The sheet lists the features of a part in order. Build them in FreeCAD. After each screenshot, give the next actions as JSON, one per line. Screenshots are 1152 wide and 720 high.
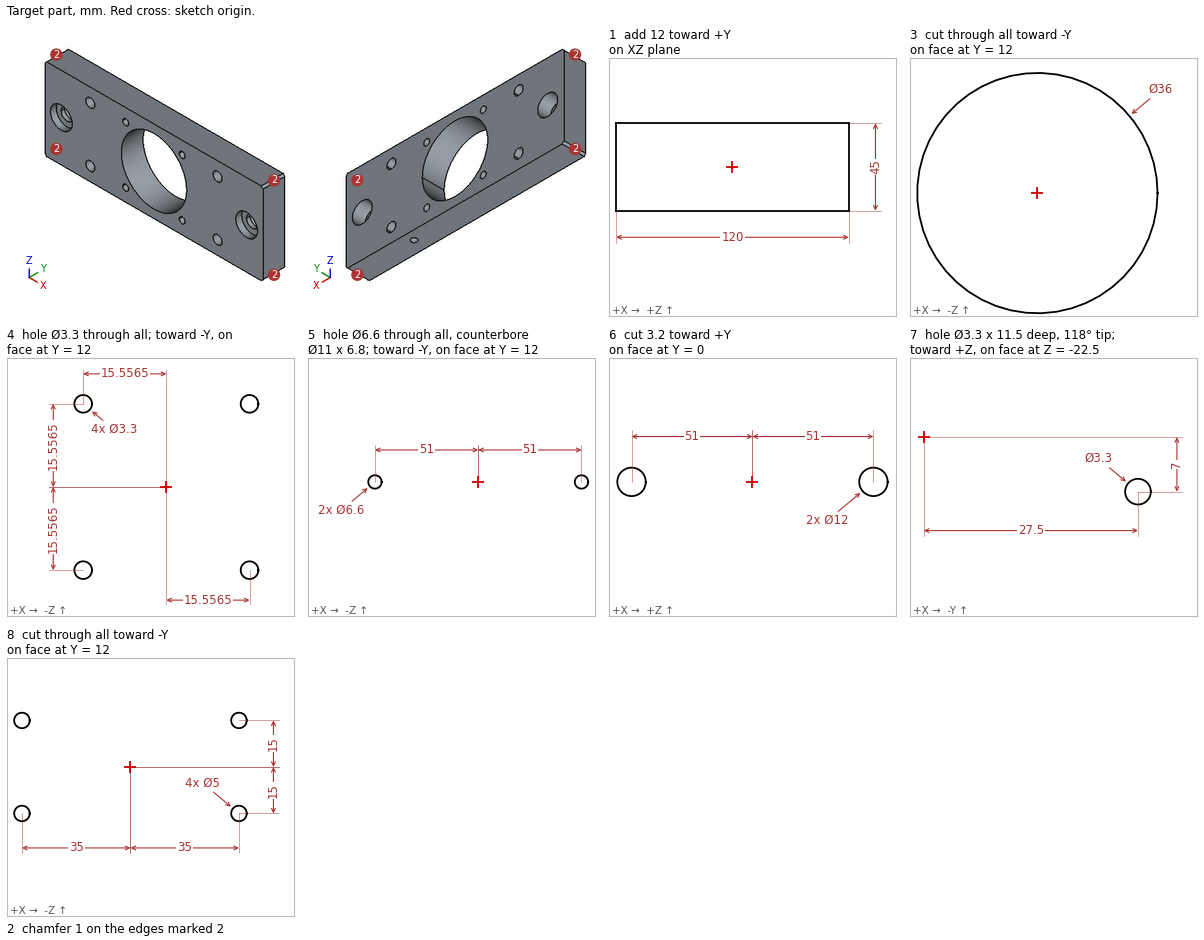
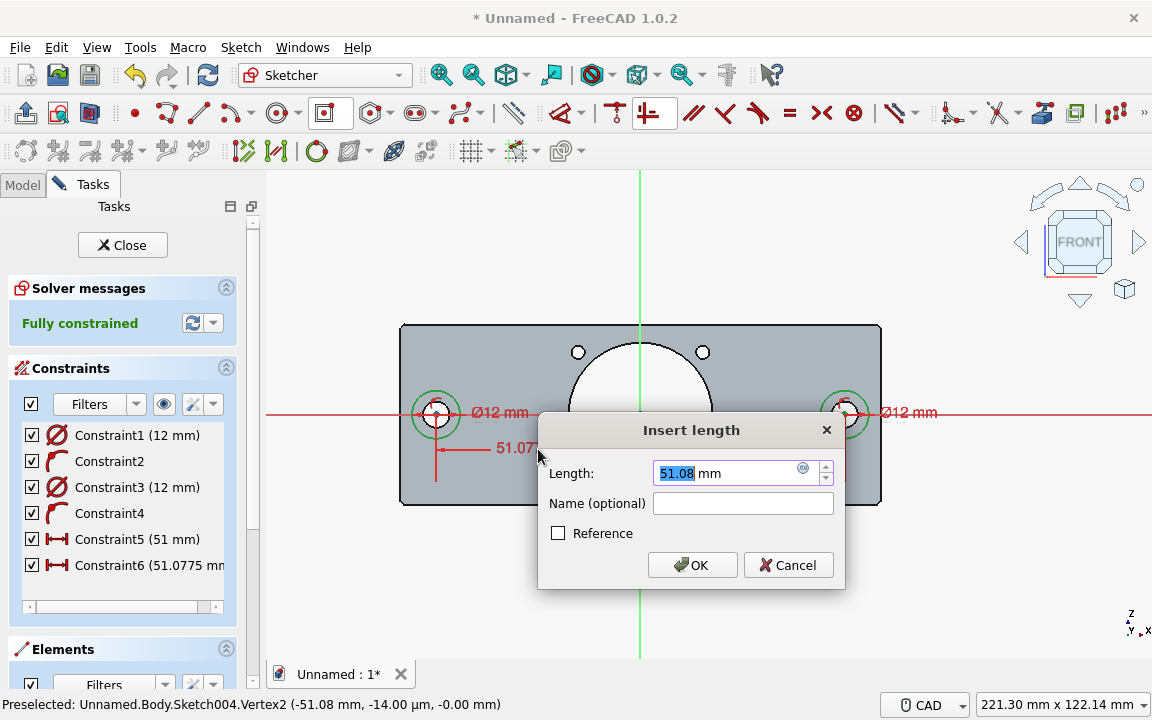
{"action": "type", "text": "51"}
{"action": "key", "text": "Return"}
{"action": "key", "text": "Escape"}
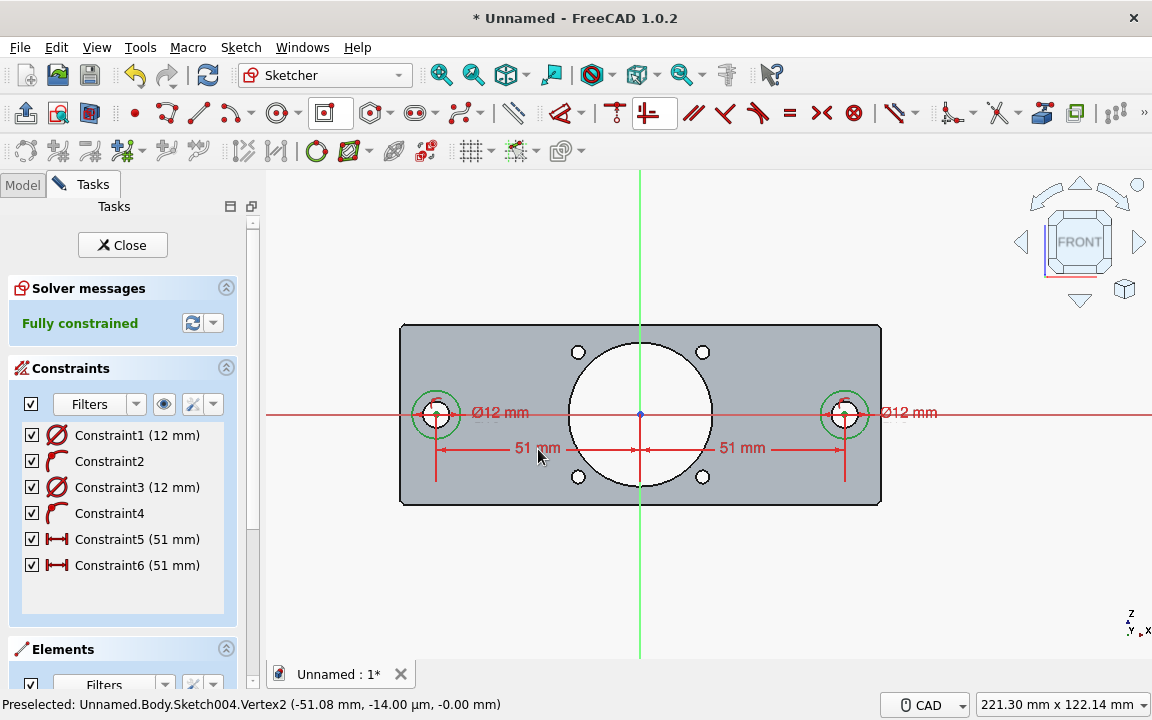
{"action": "left_click", "coordinate": [123, 245]}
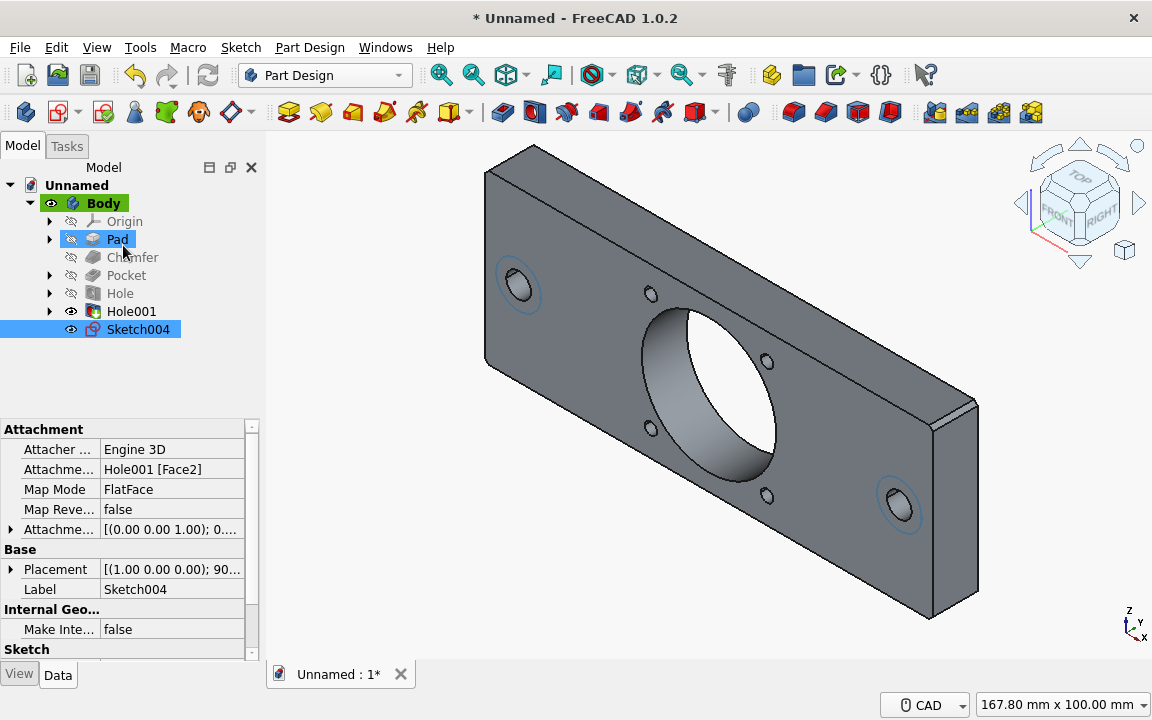
{"action": "left_click", "coordinate": [504, 112]}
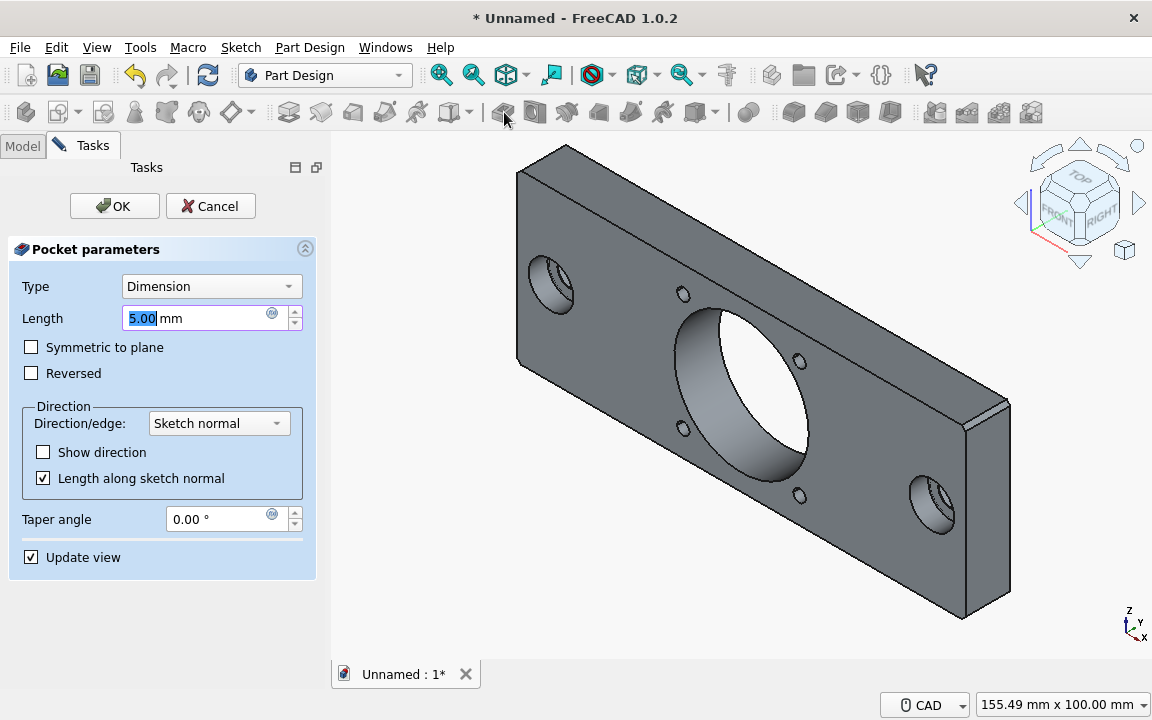
{"action": "type", "text": "3.2"}
{"action": "key", "text": "Tab"}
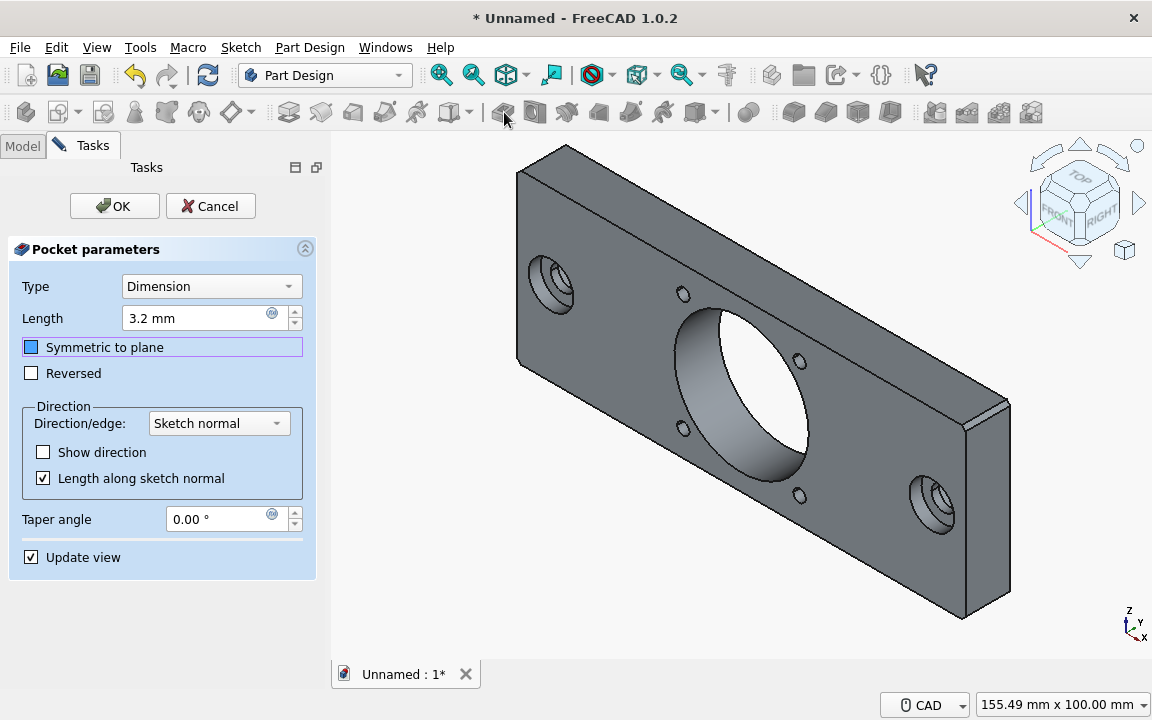
{"action": "left_click", "coordinate": [115, 206]}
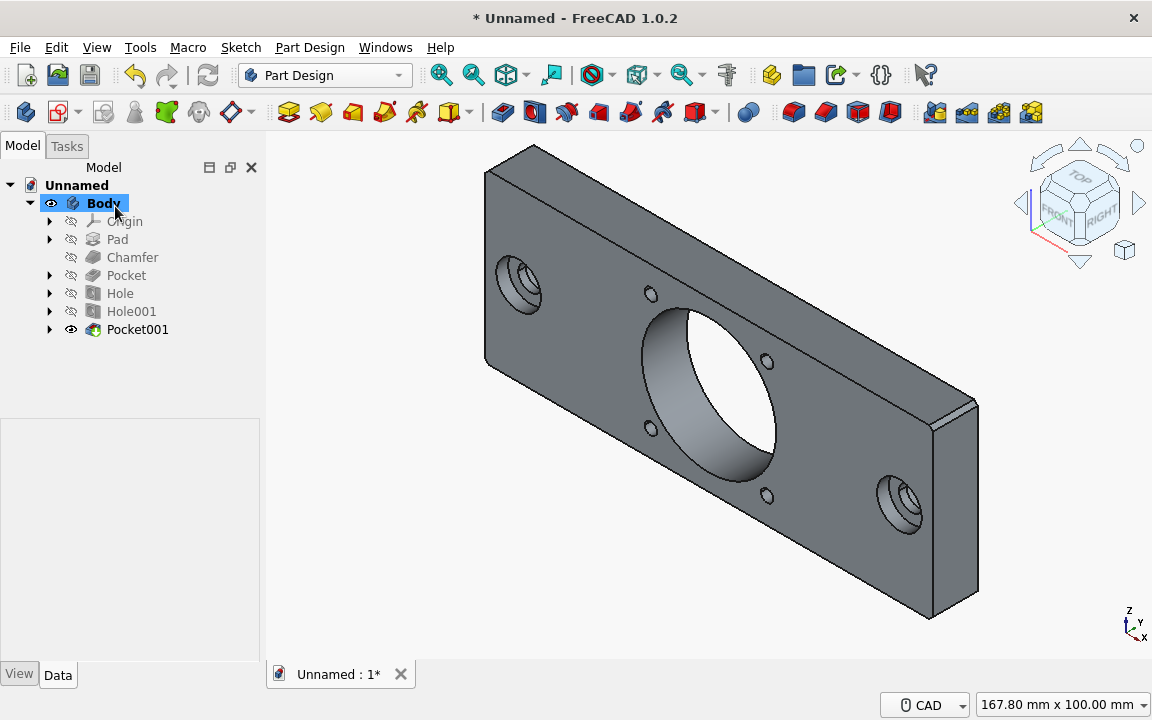
{"action": "key", "text": "5"}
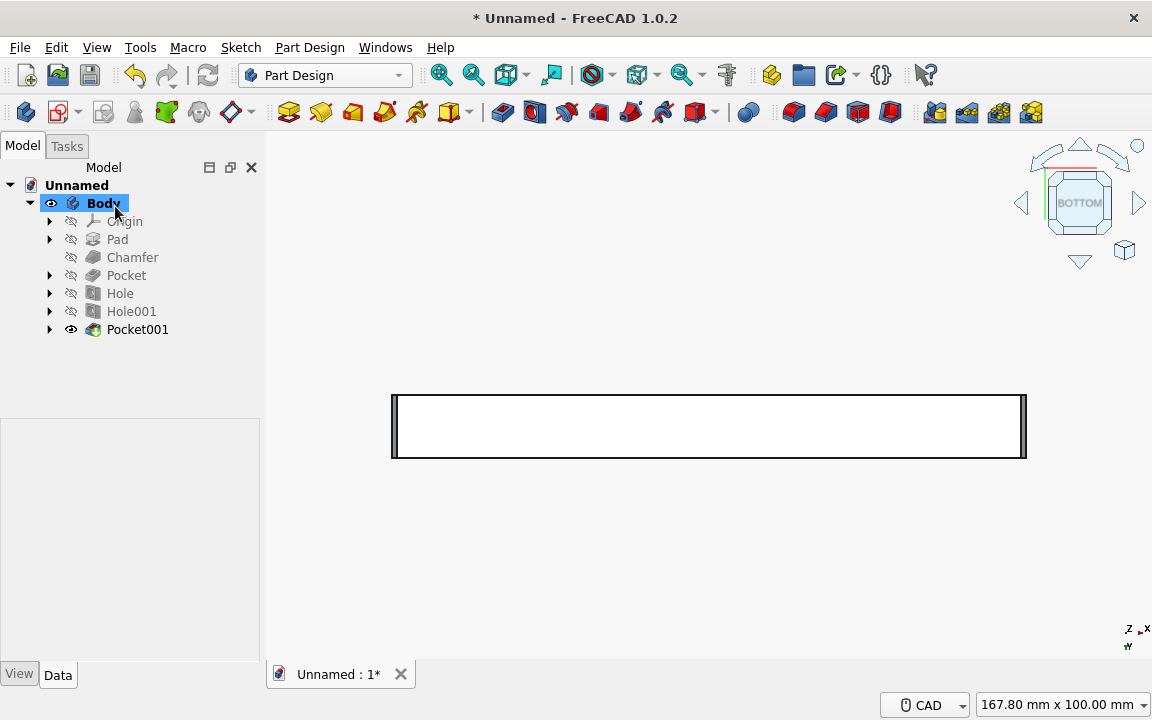
{"action": "left_click", "coordinate": [976, 426]}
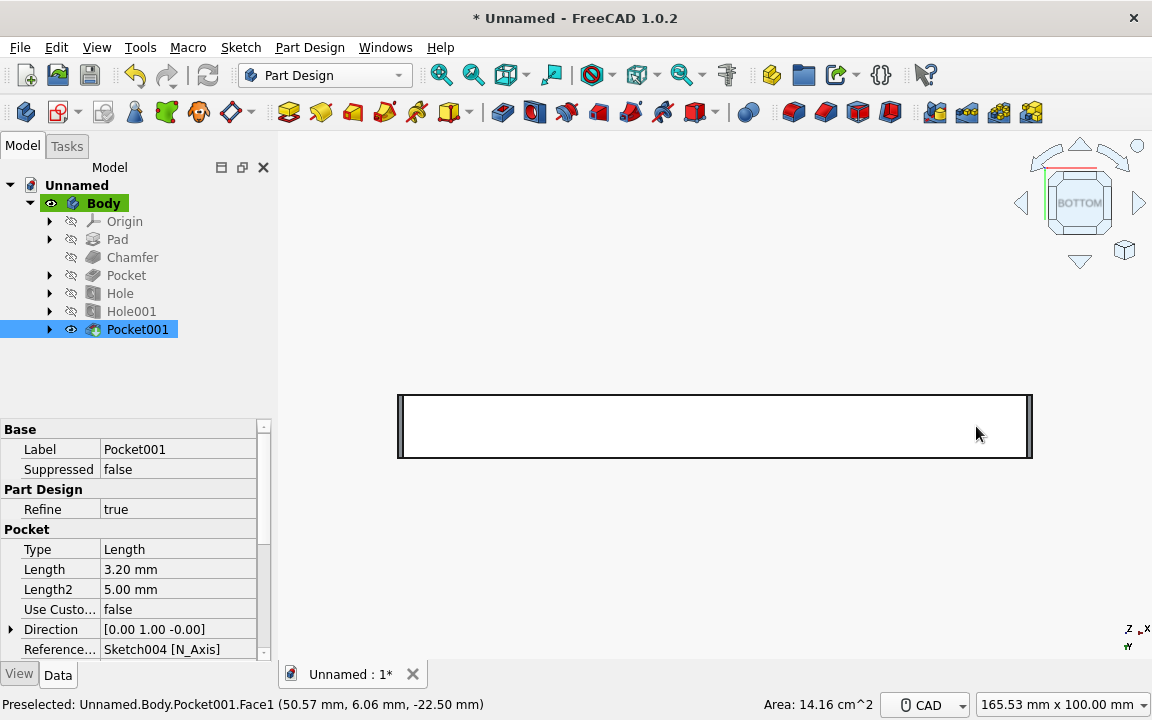
{"action": "left_click", "coordinate": [58, 112]}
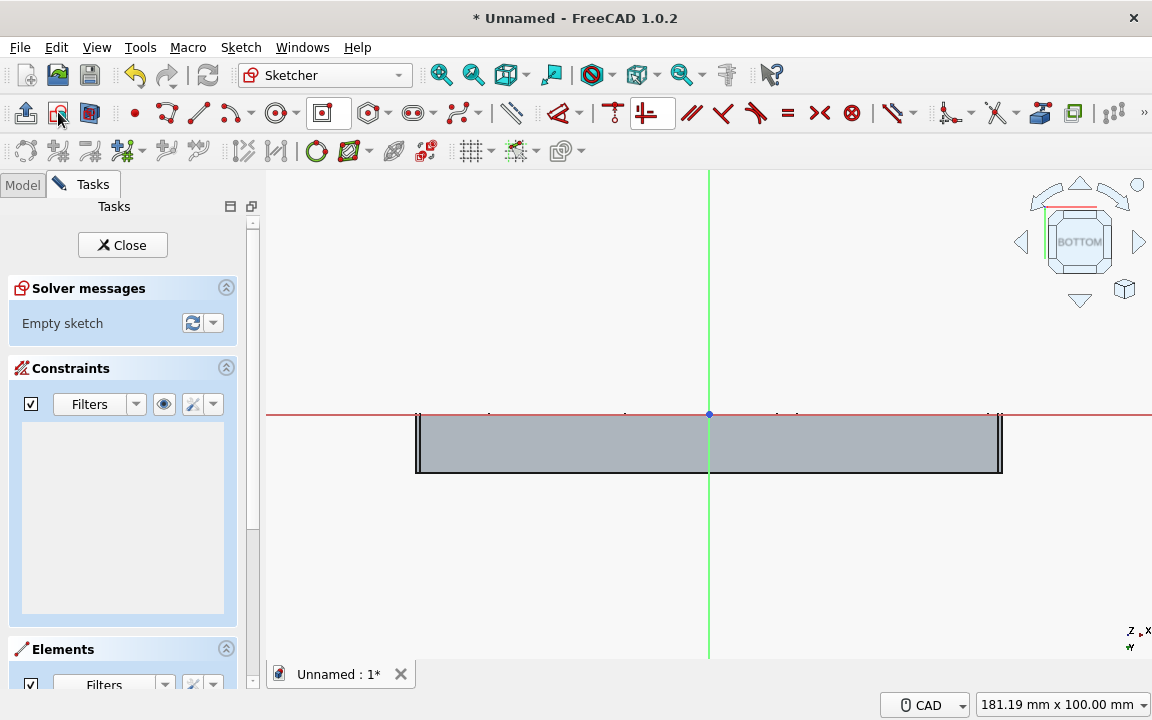
{"action": "scroll", "coordinate": [854, 451], "scroll_direction": "up", "scroll_amount": 15}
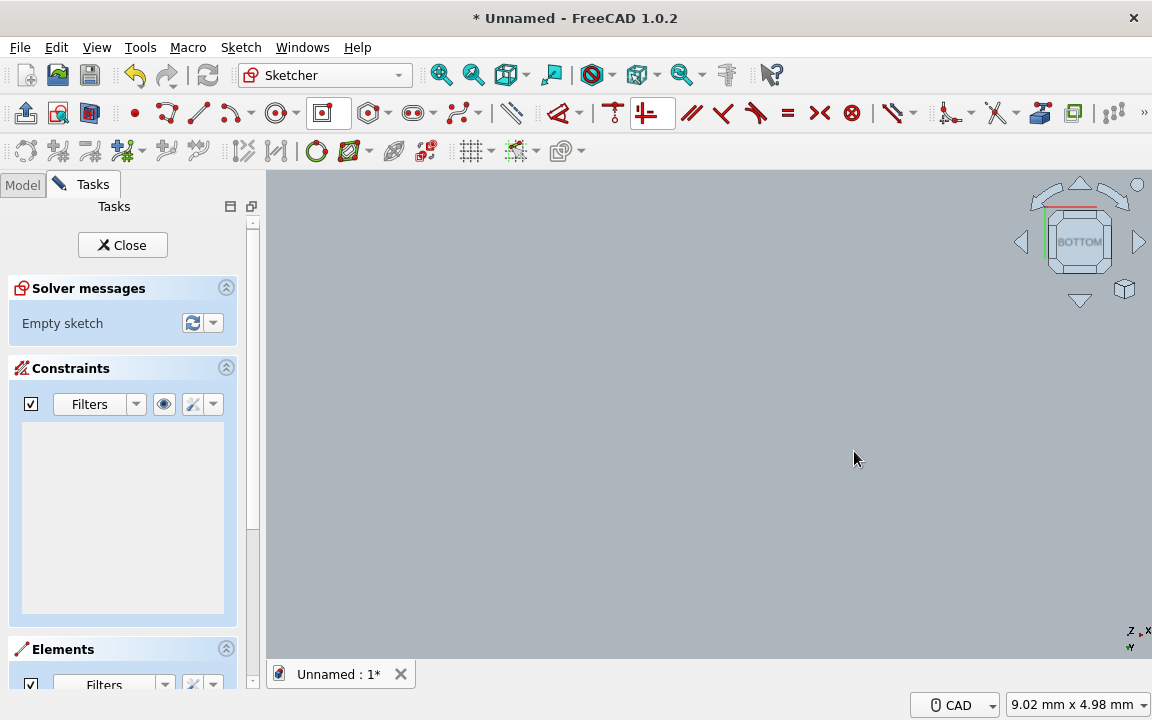
{"action": "left_click", "coordinate": [276, 114]}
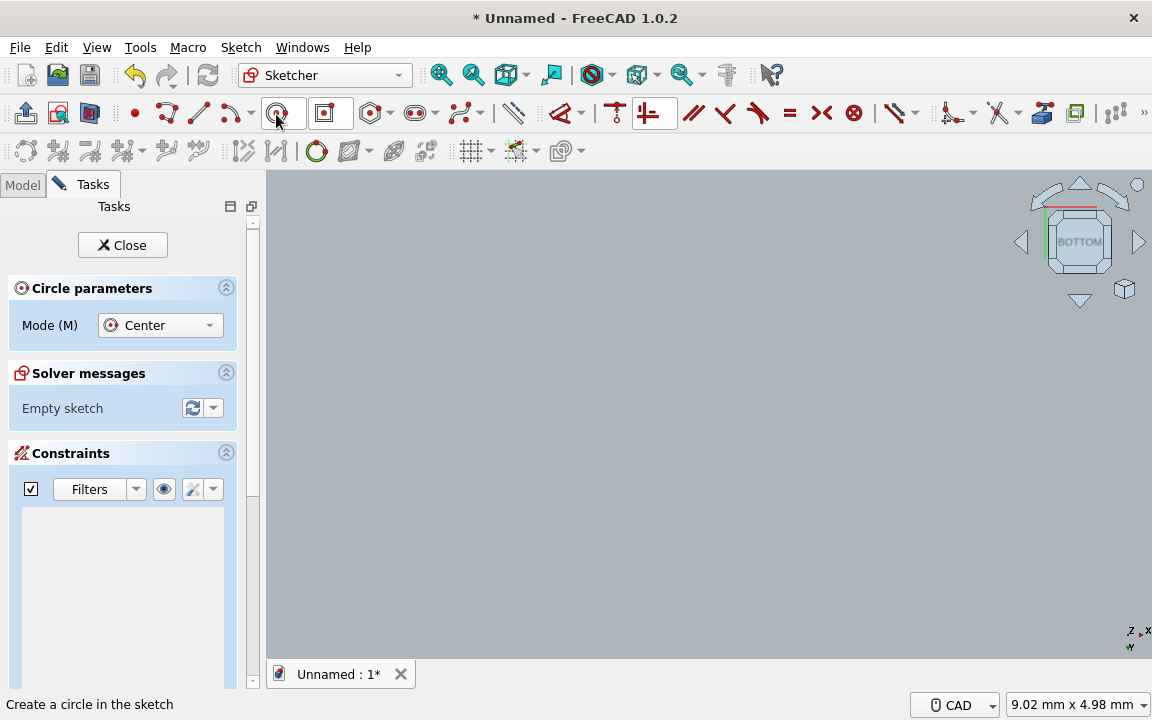
{"action": "left_click", "coordinate": [630, 394]}
{"action": "mouse_move", "coordinate": [745, 280]}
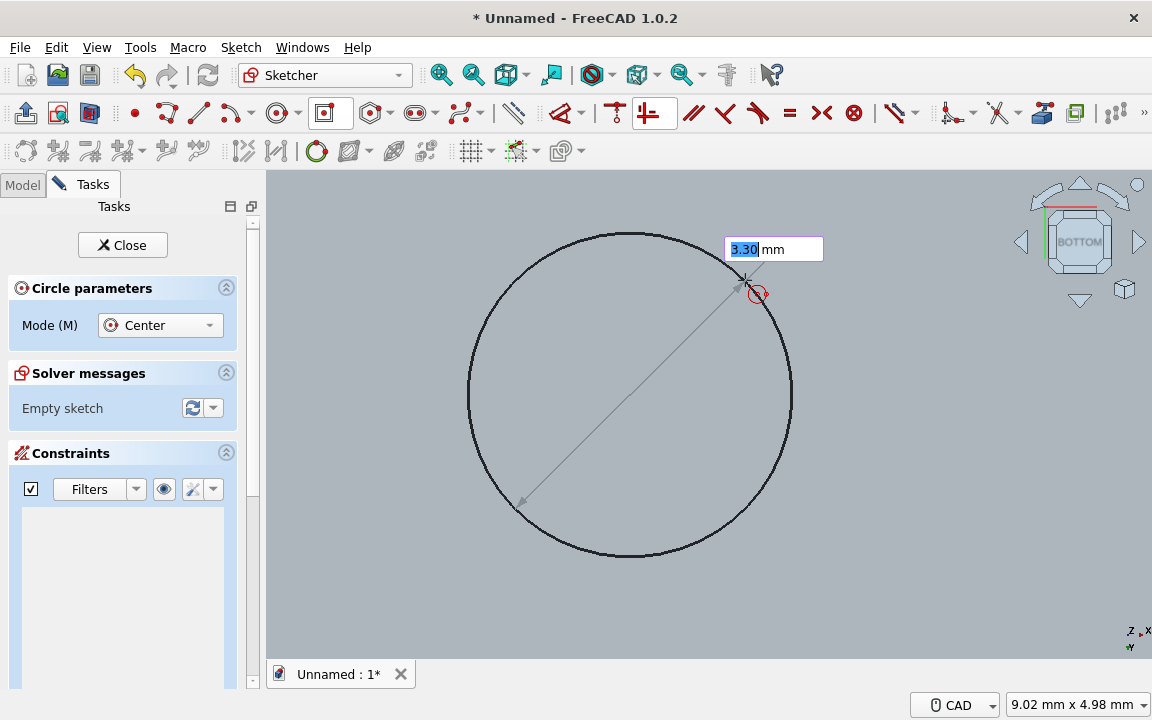
{"action": "type", "text": "3.3"}
{"action": "key", "text": "Return"}
{"action": "key", "text": "Escape"}